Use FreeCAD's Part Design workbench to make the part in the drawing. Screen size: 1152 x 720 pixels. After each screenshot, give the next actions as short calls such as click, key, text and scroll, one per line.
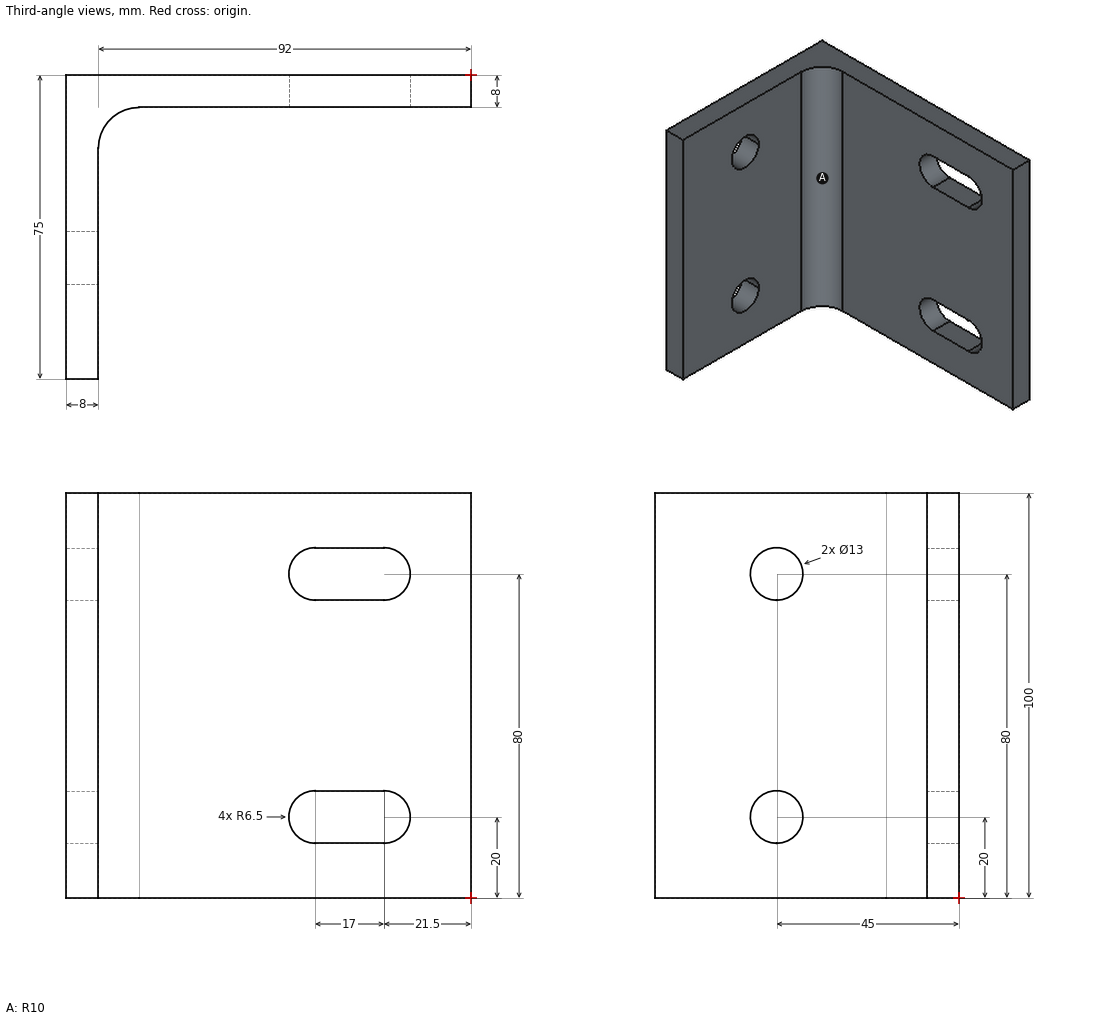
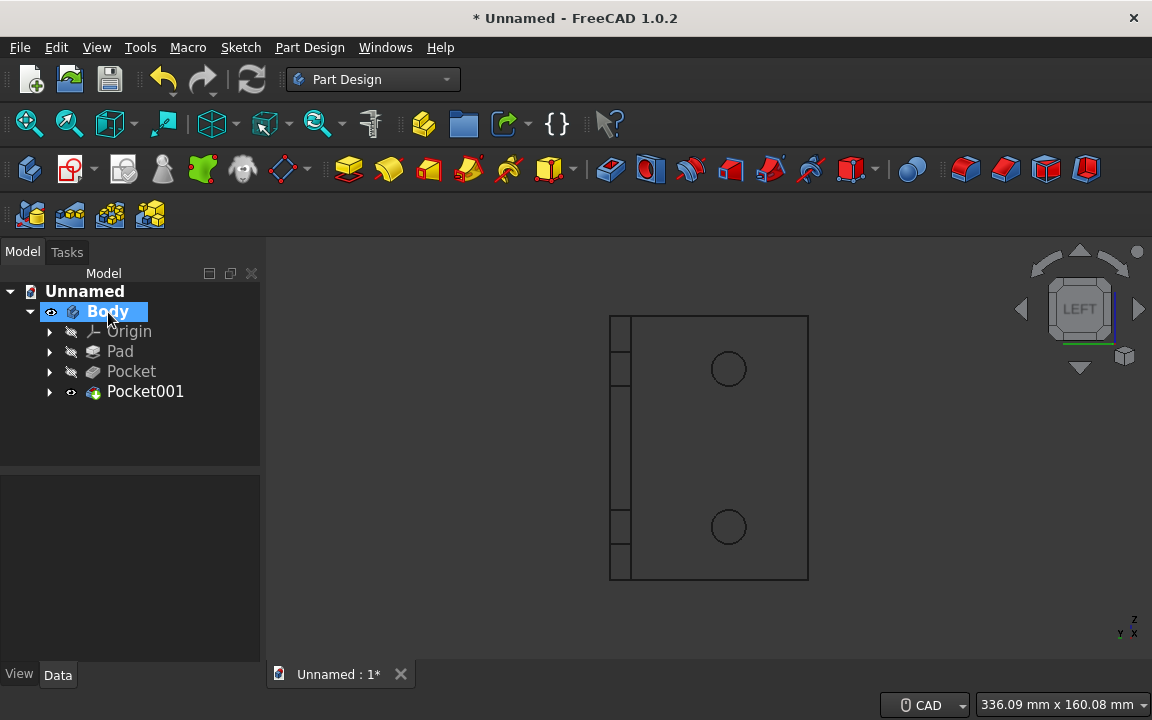
key(0)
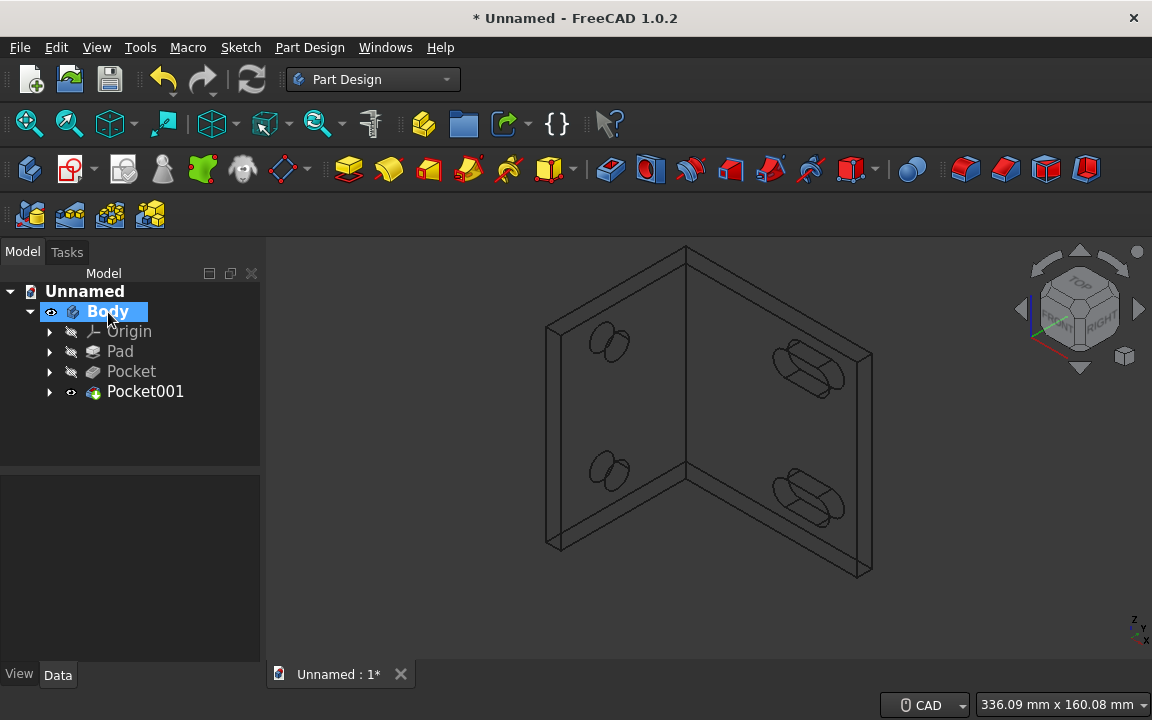
click(686, 370)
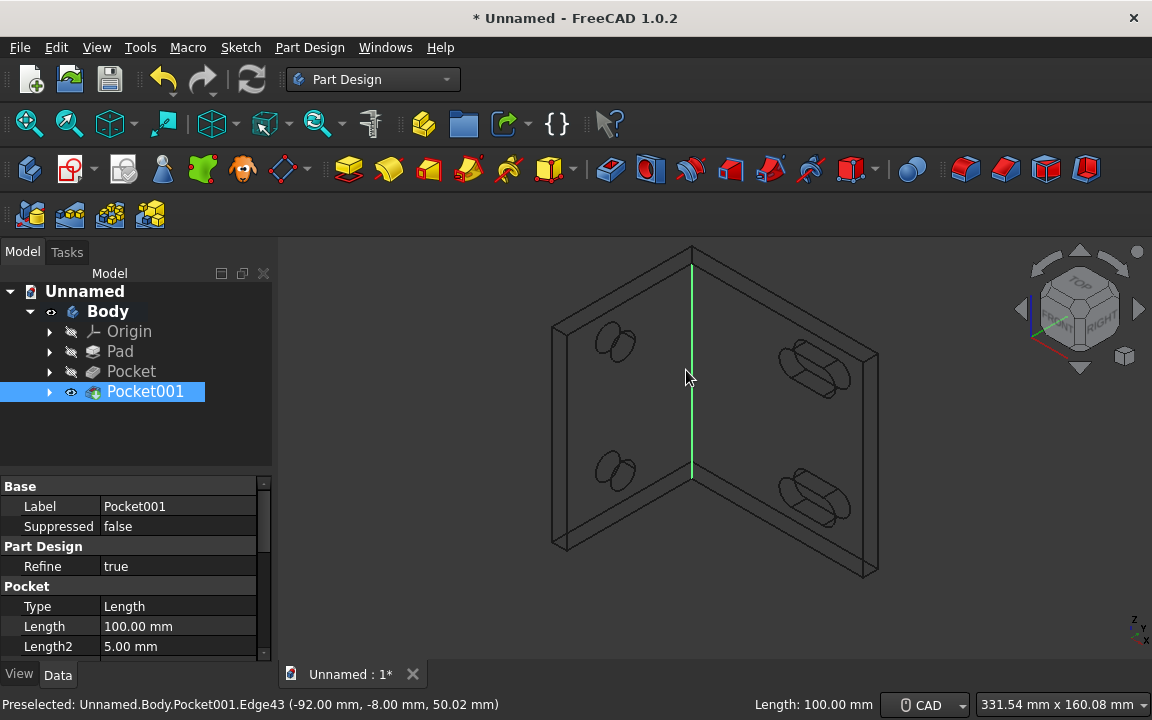
key(v)
key(1)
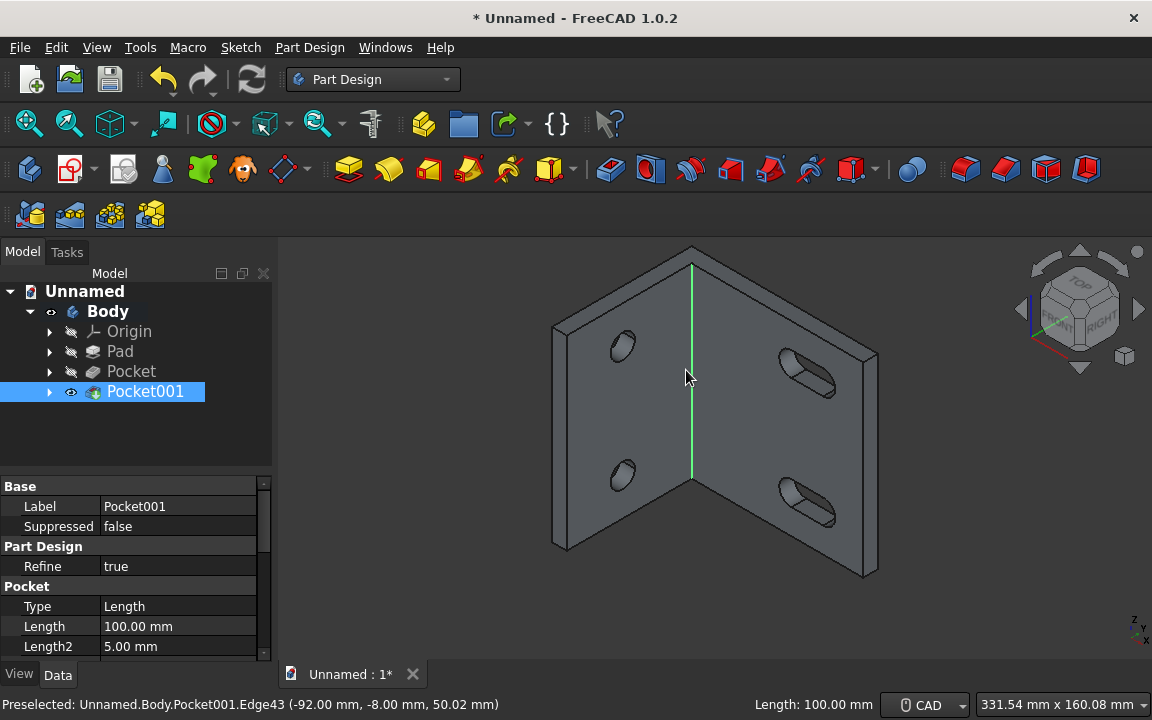
click(966, 170)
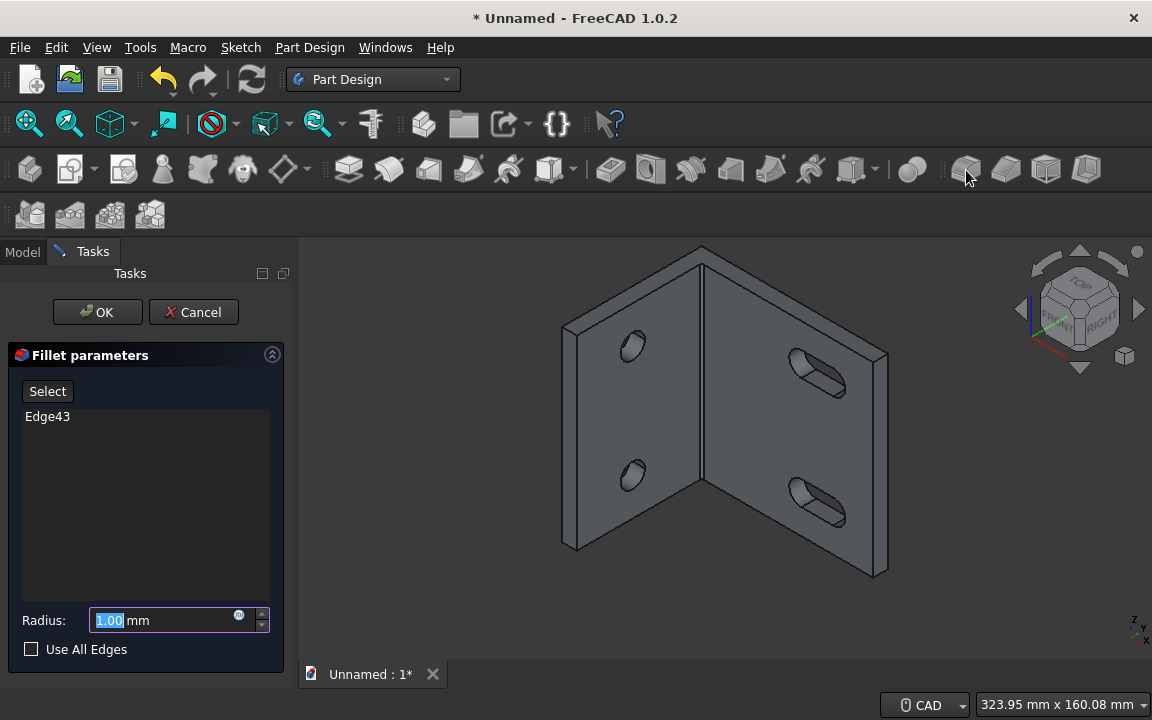
text(10)
key(Tab)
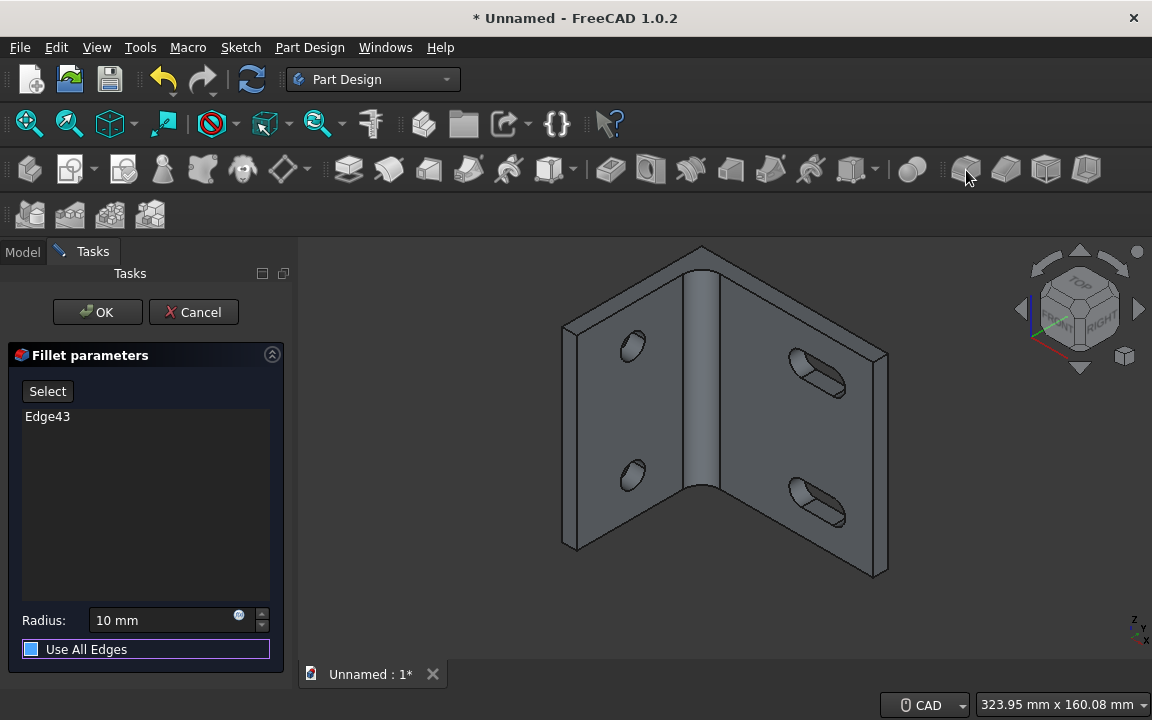
click(98, 312)